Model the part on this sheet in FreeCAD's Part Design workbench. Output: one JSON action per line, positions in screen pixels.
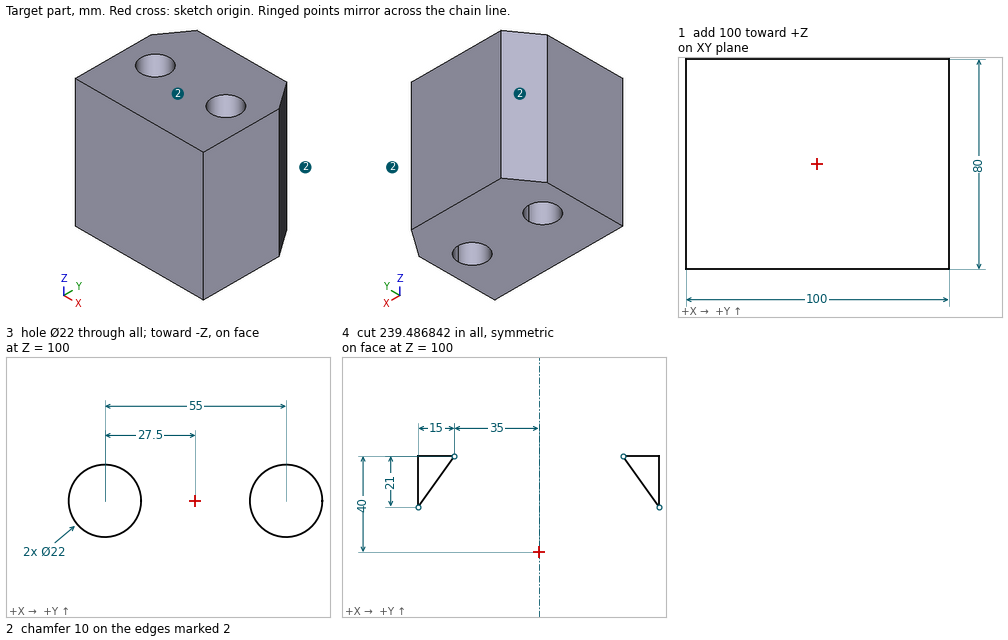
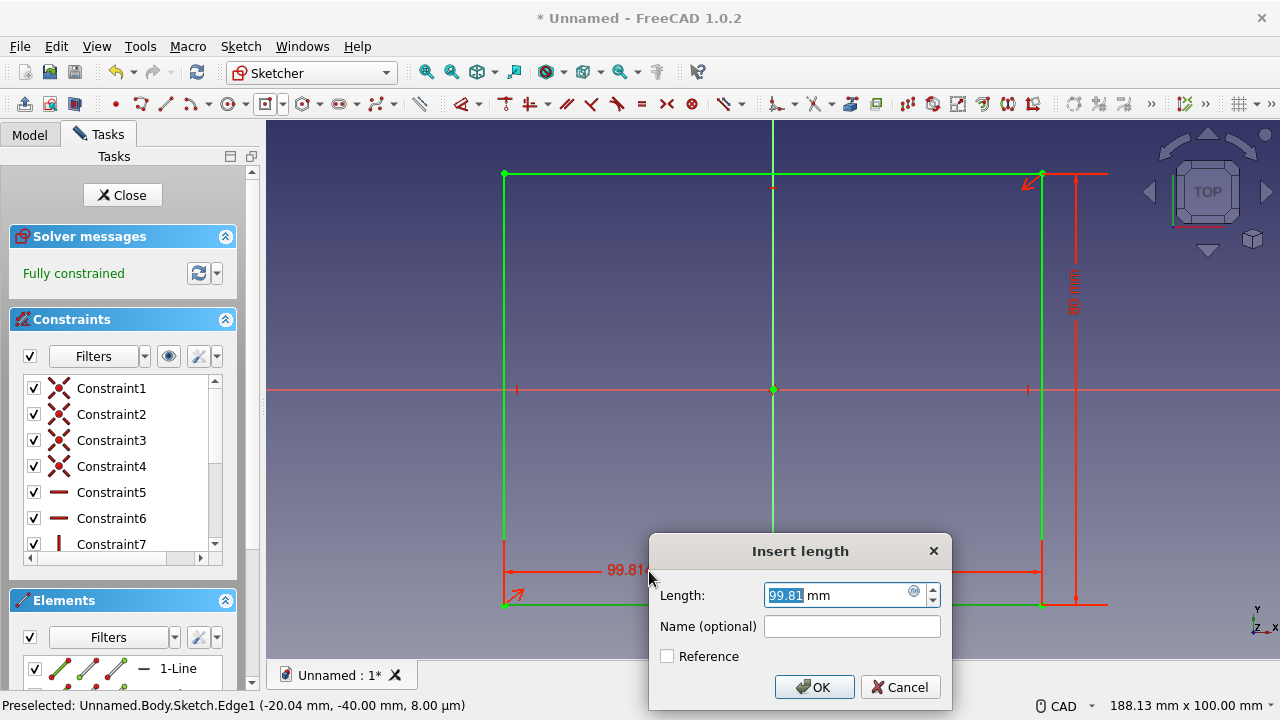
{"action": "type", "text": "100"}
{"action": "key", "text": "Return"}
{"action": "key", "text": "Escape"}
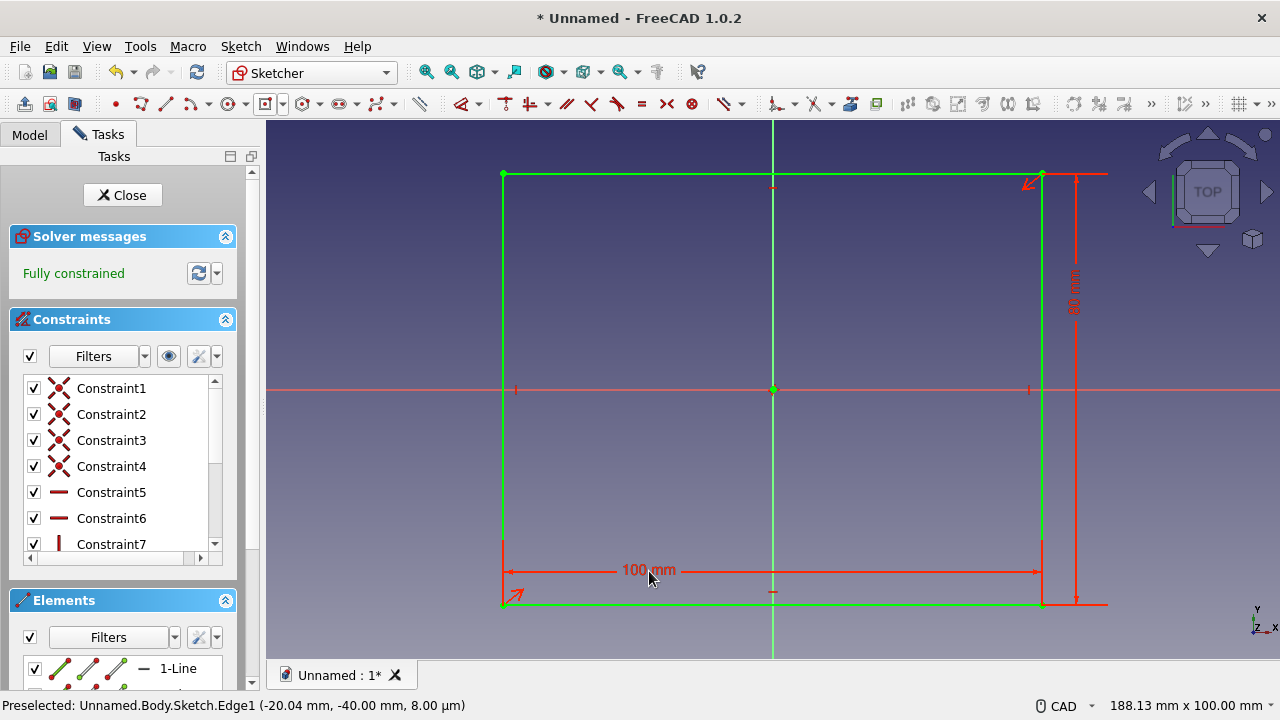
{"action": "left_click", "coordinate": [123, 195]}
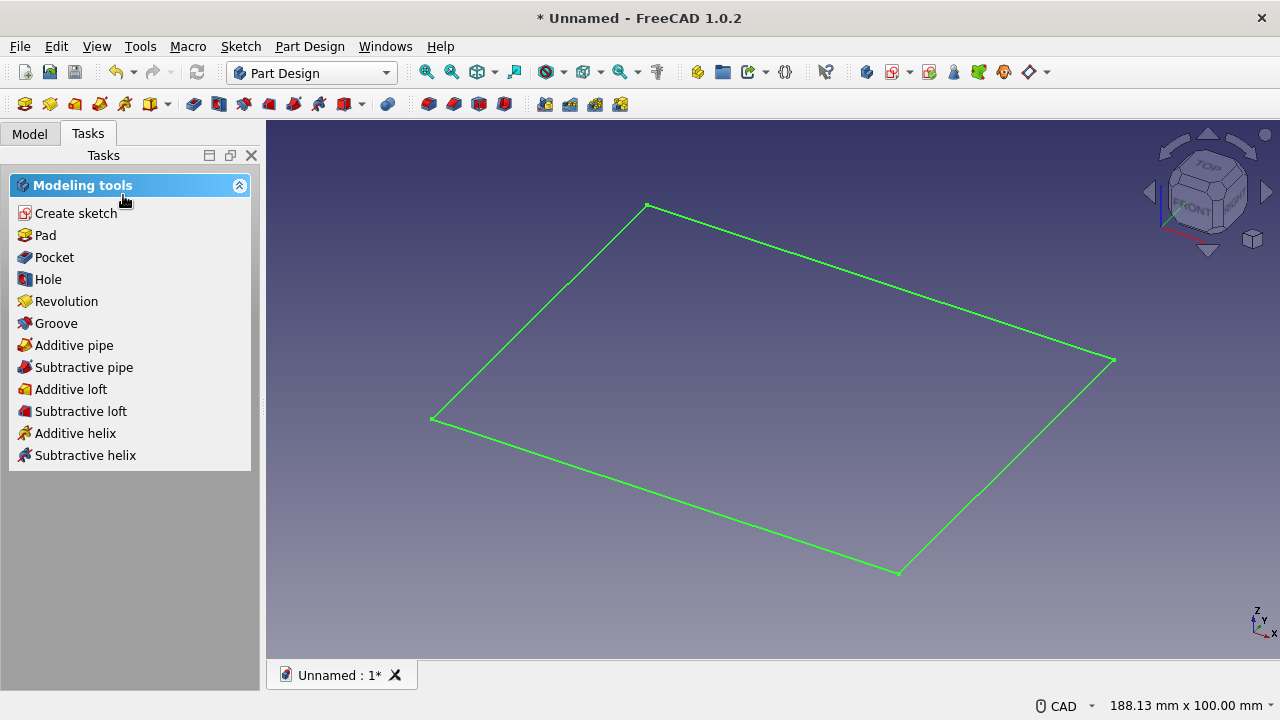
{"action": "left_click", "coordinate": [25, 104]}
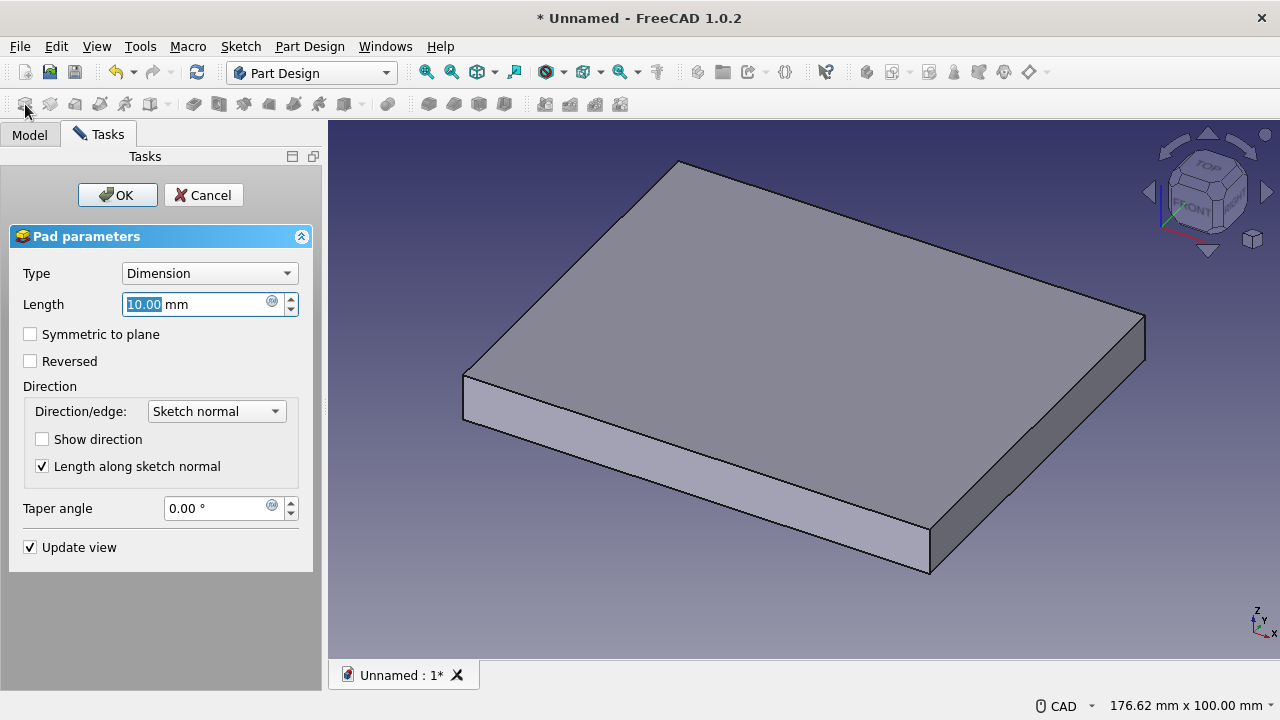
{"action": "type", "text": "100"}
{"action": "key", "text": "Tab"}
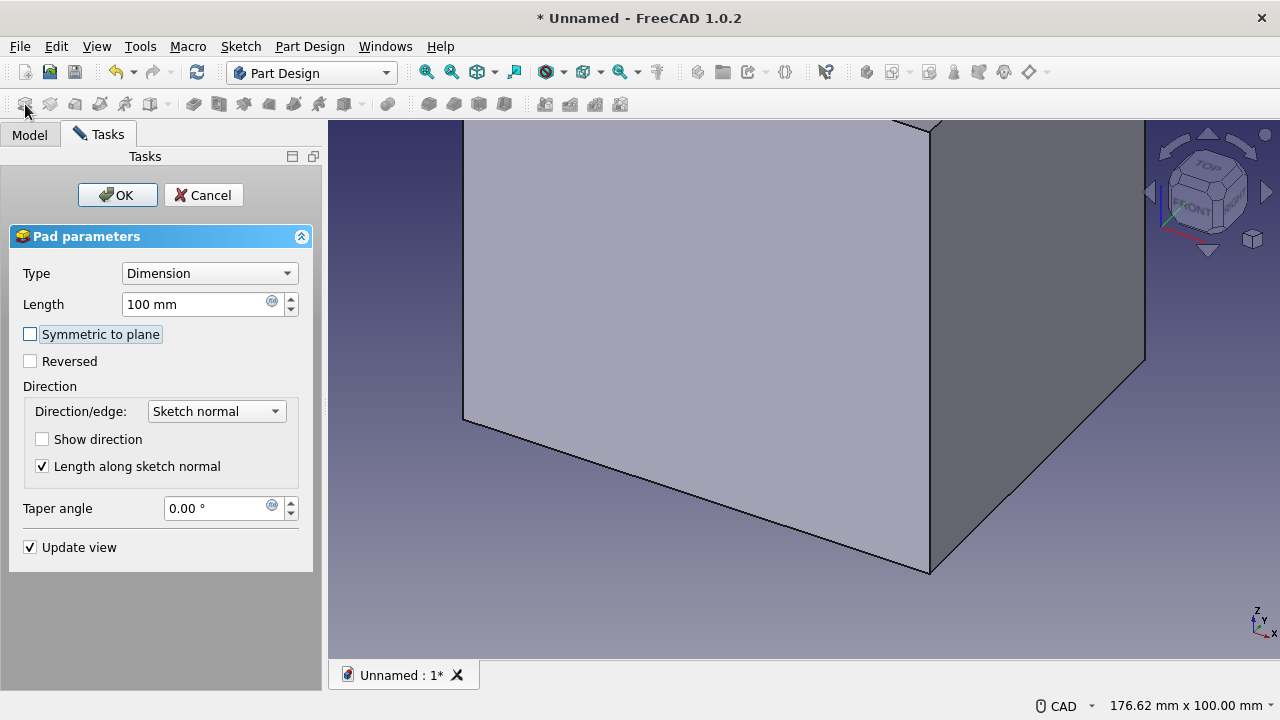
{"action": "left_click", "coordinate": [118, 195]}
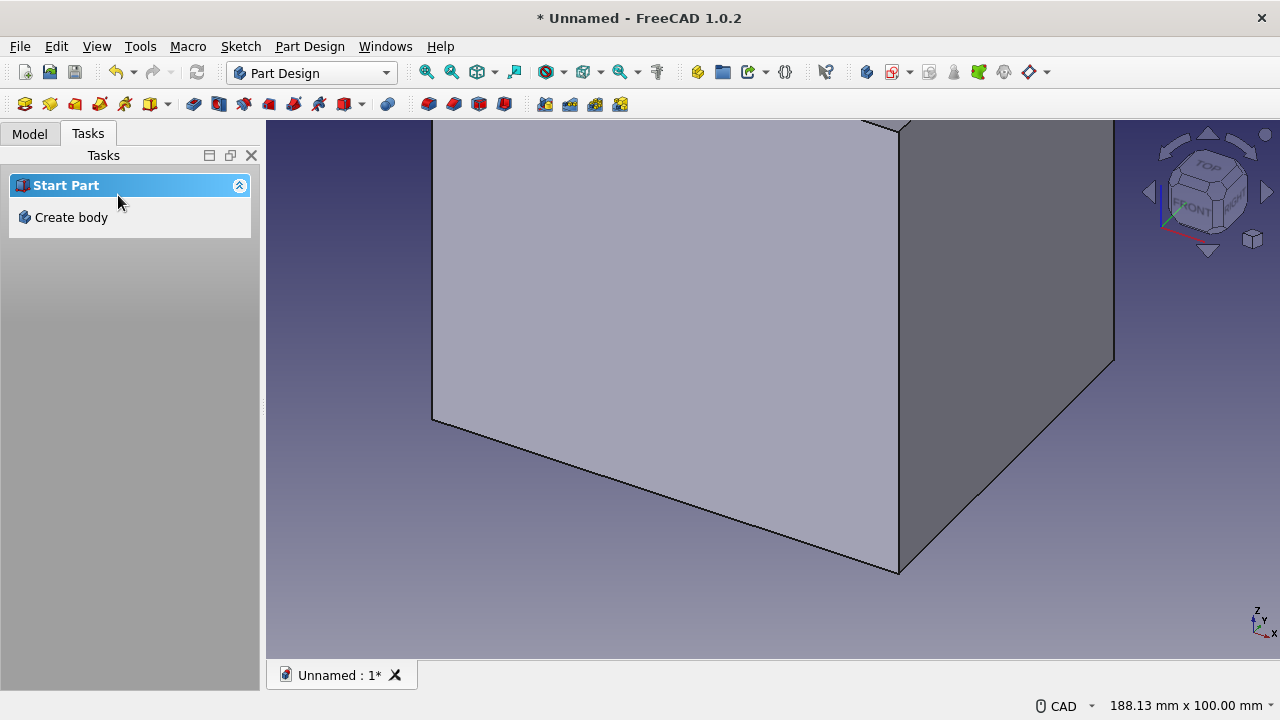
{"action": "left_click", "coordinate": [427, 72]}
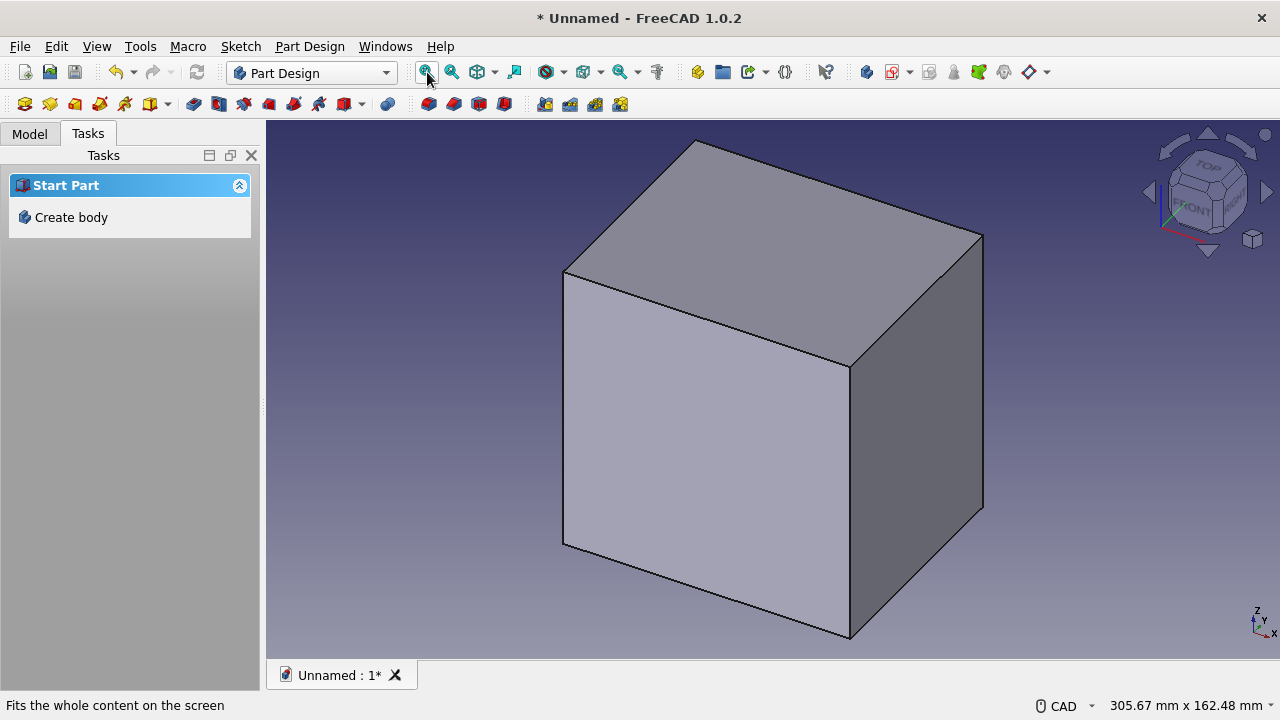
{"action": "key", "text": "0"}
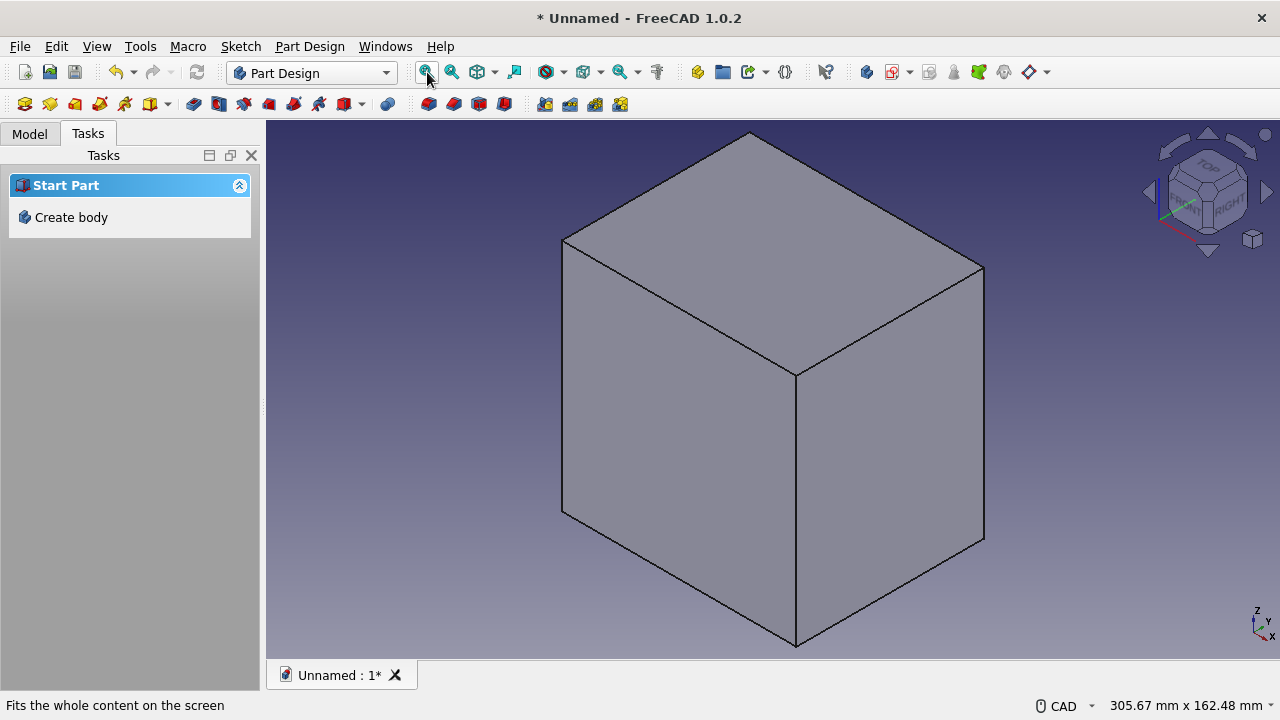
{"action": "key", "text": "2"}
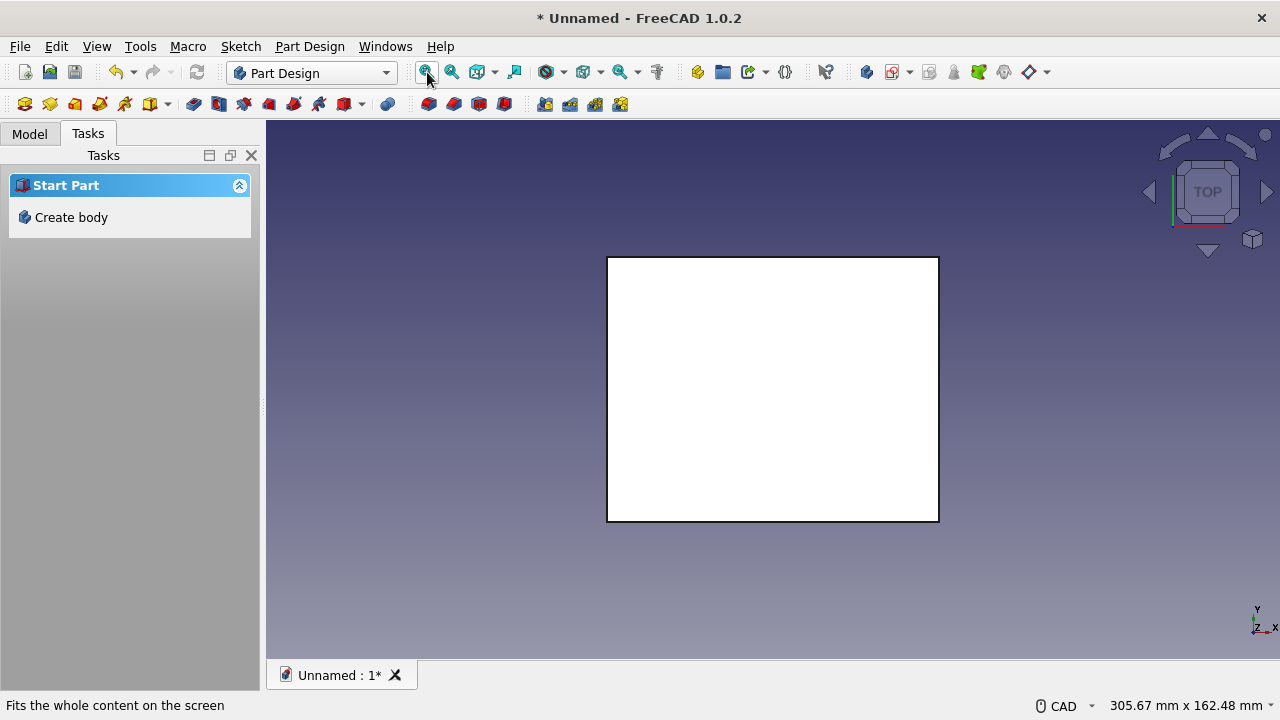
{"action": "key", "text": "1"}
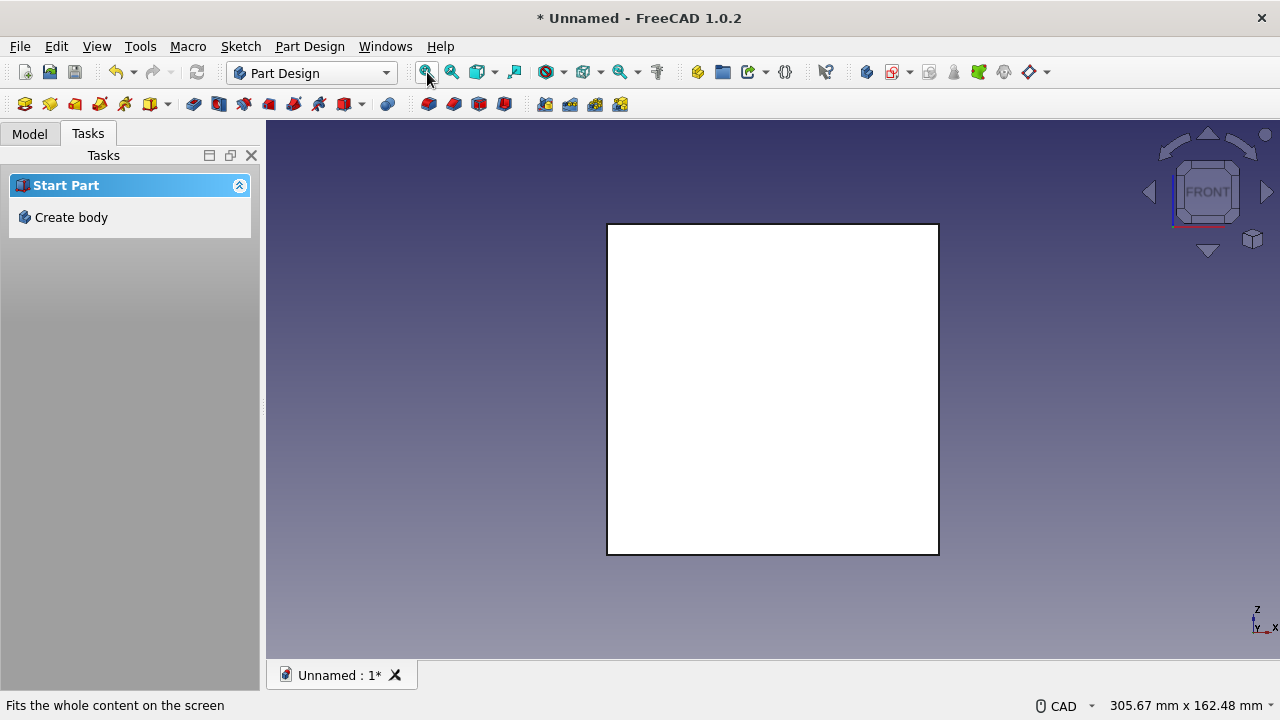
{"action": "key", "text": "3"}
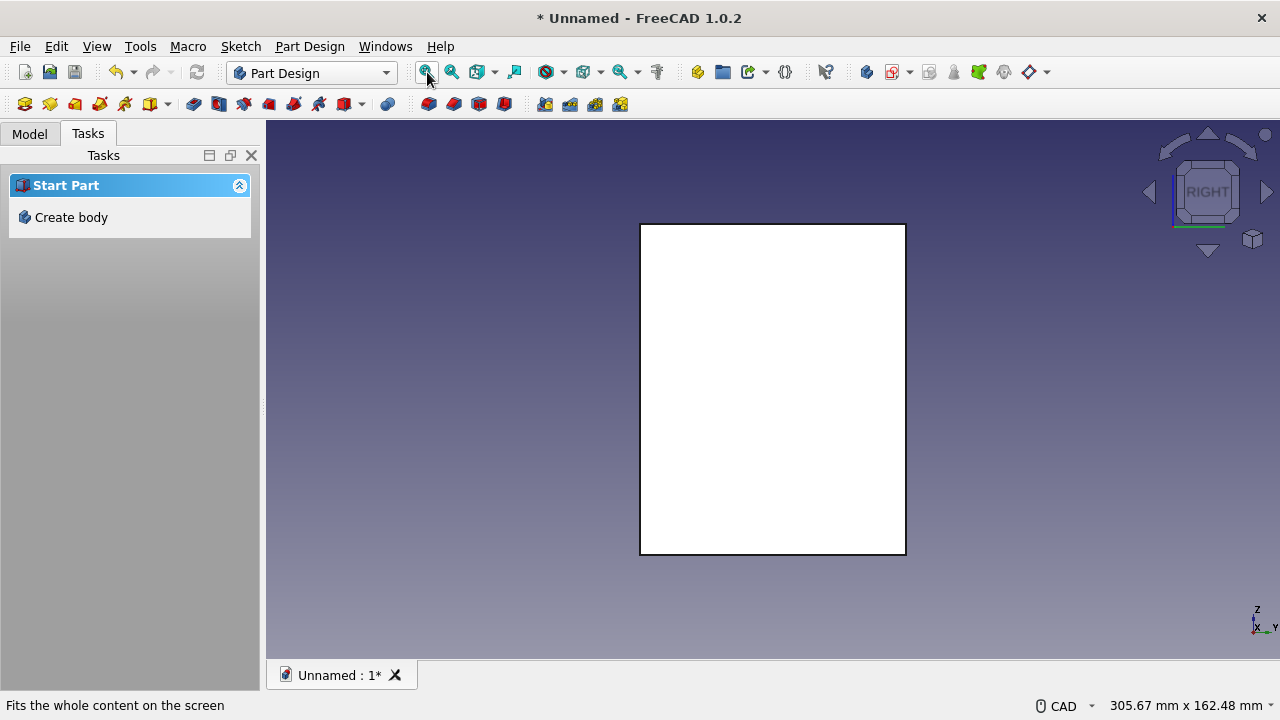
{"action": "left_click", "coordinate": [906, 388]}